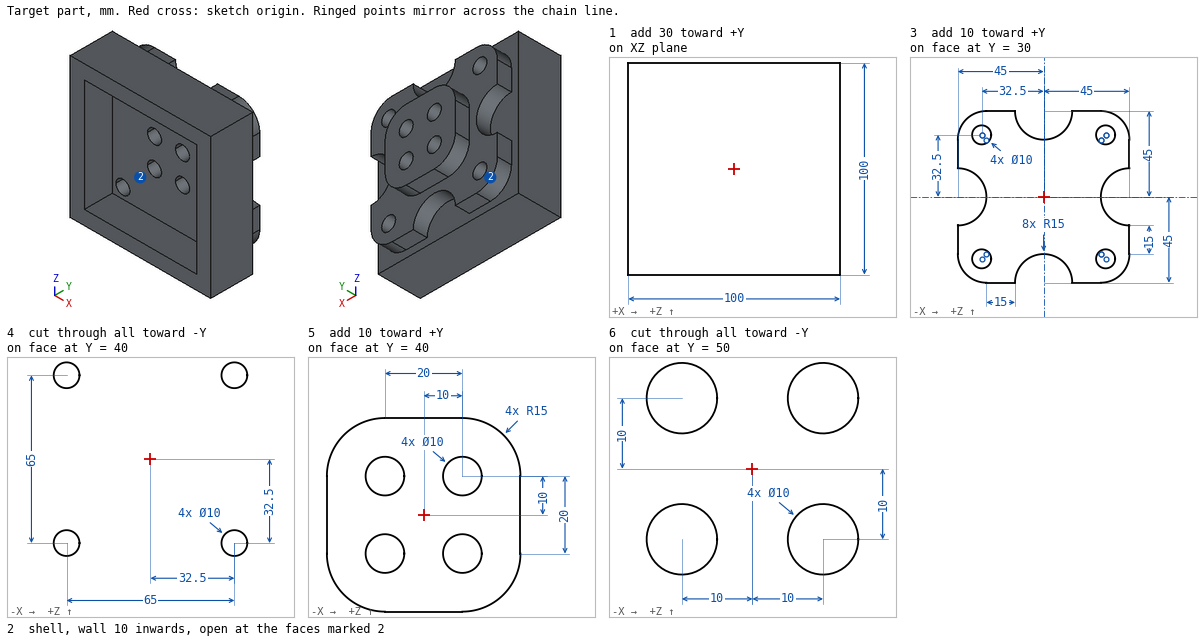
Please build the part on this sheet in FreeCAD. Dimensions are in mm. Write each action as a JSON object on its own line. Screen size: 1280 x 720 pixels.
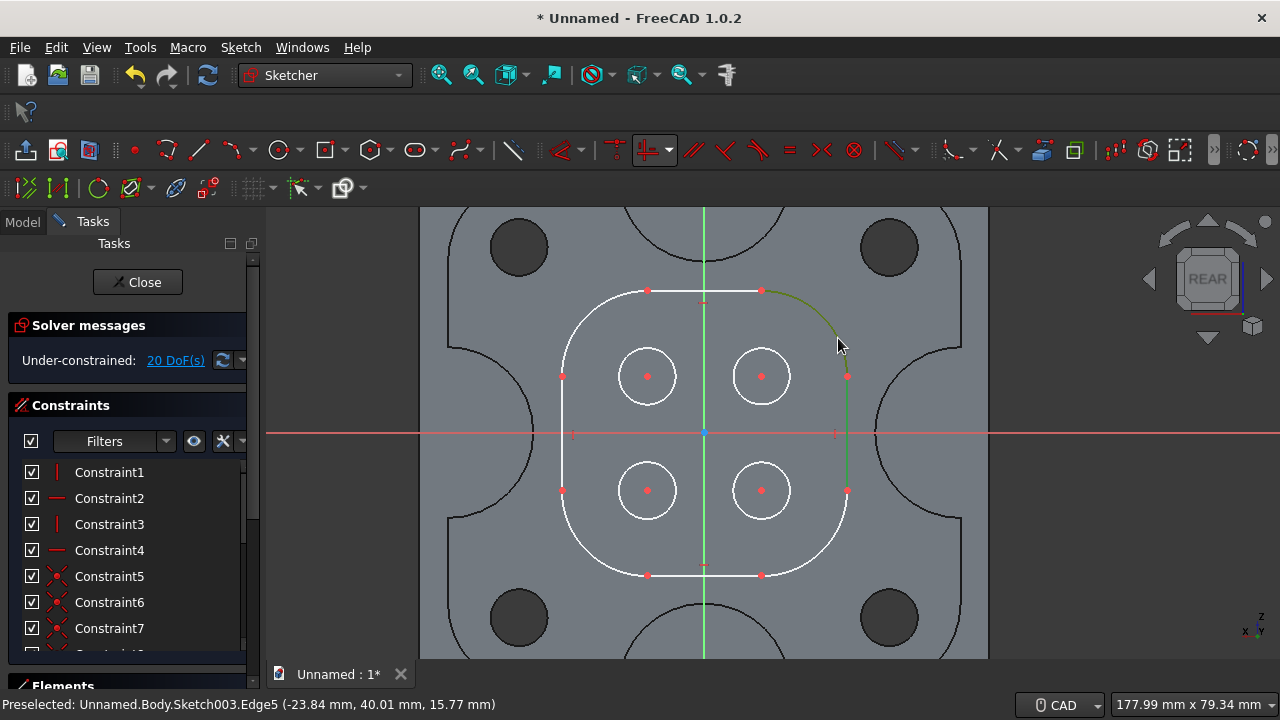
{"action": "left_click", "coordinate": [758, 150]}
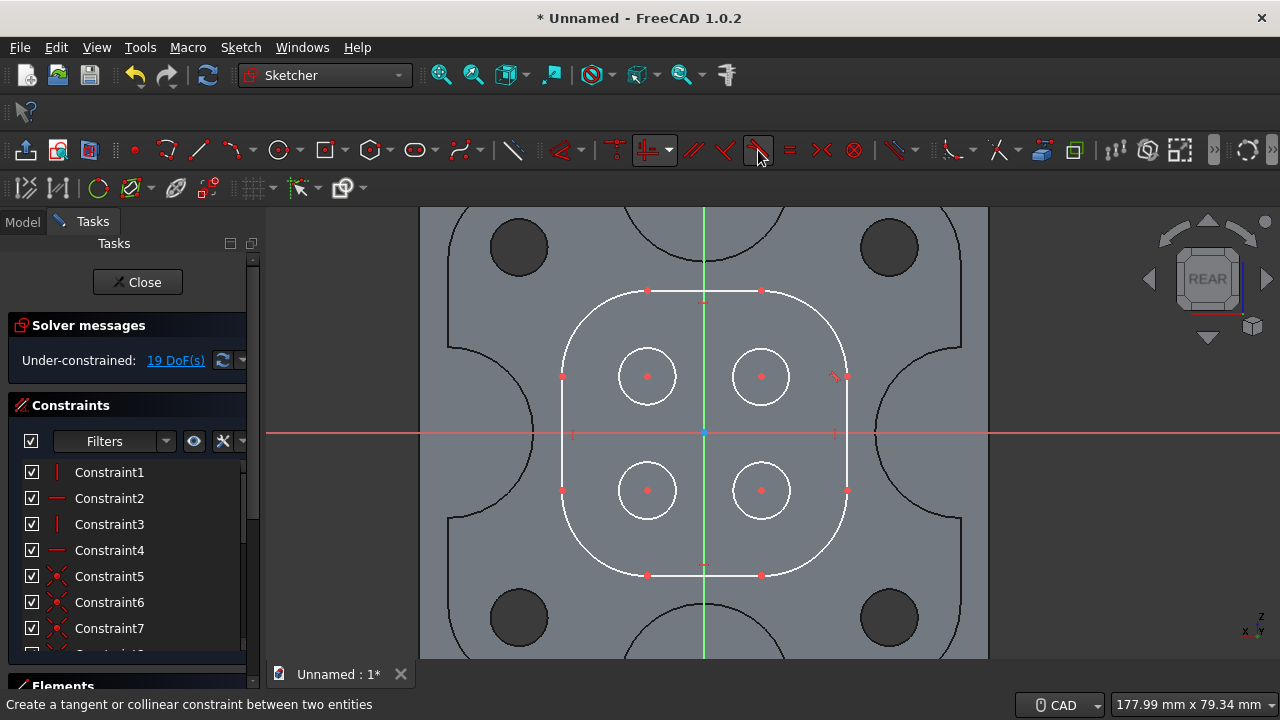
{"action": "left_click", "coordinate": [847, 457]}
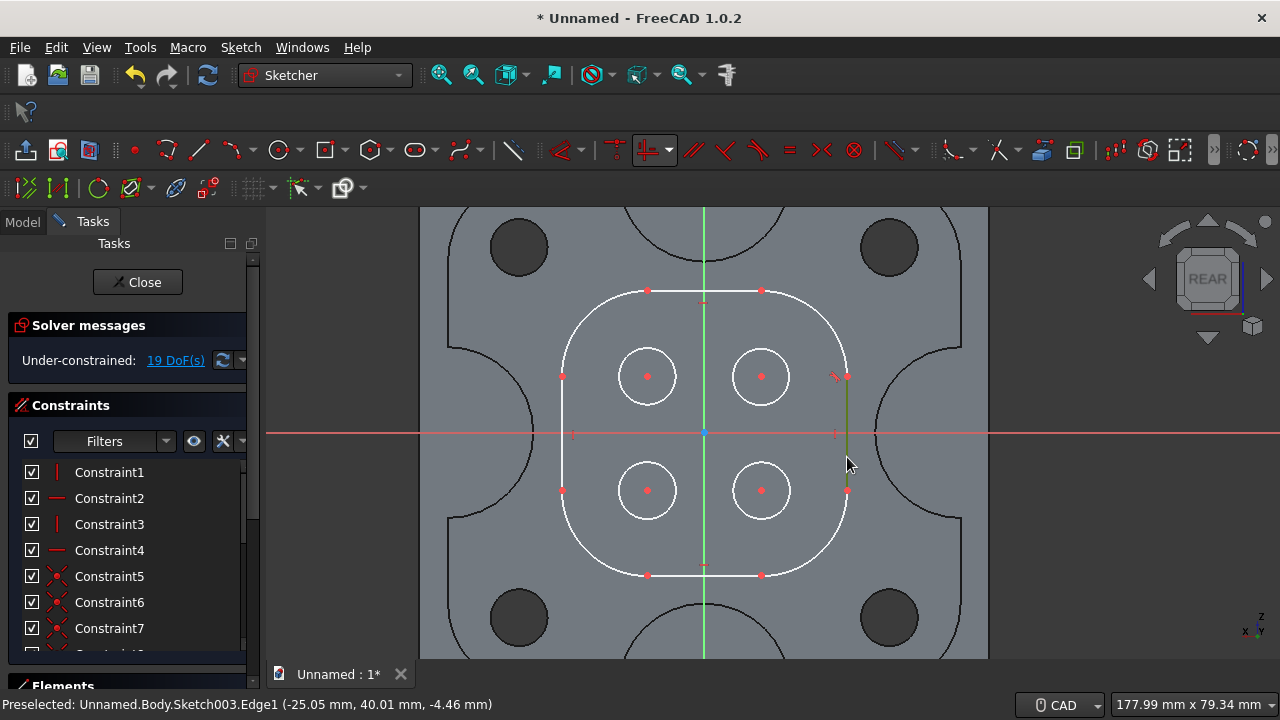
{"action": "left_click", "coordinate": [800, 567]}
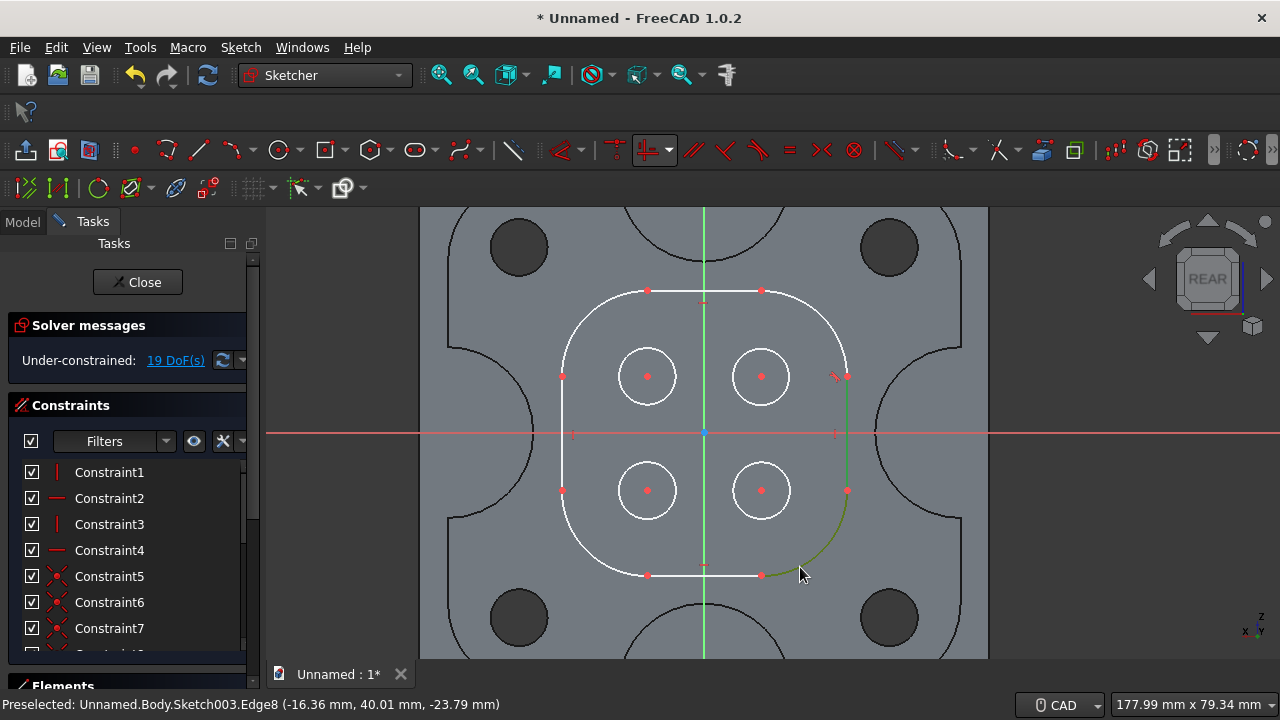
{"action": "left_click", "coordinate": [758, 150]}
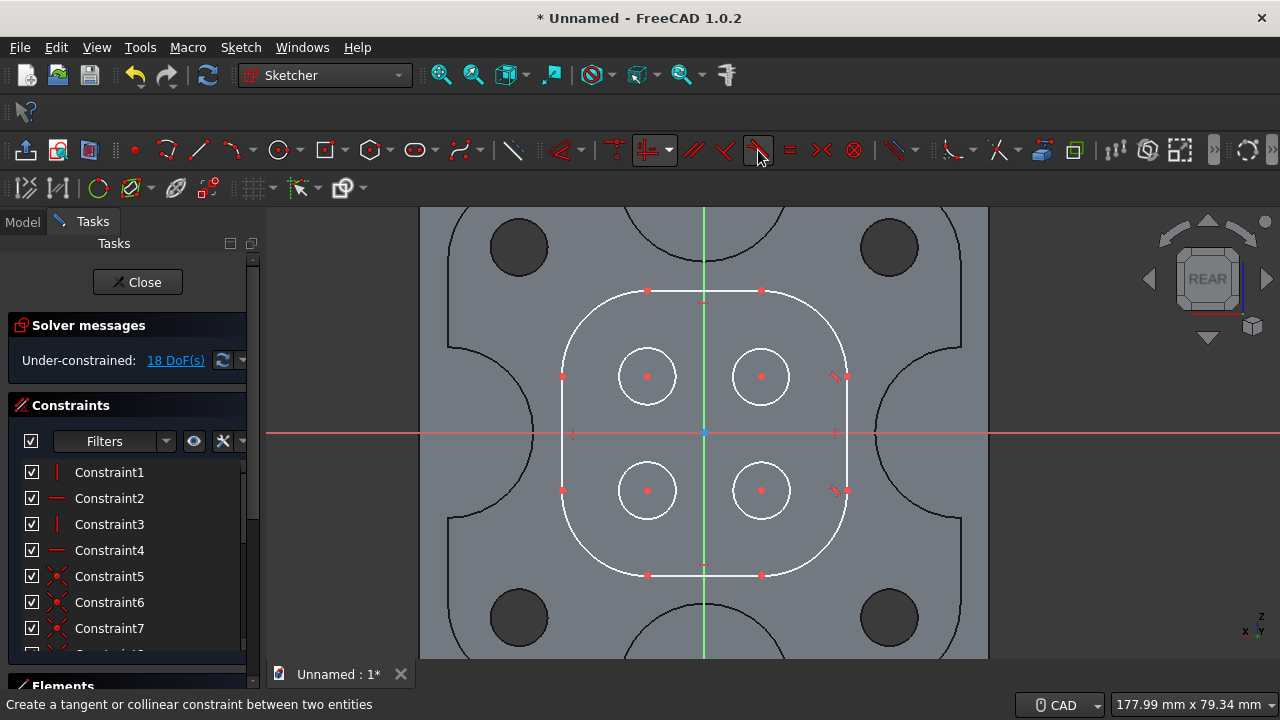
{"action": "left_click", "coordinate": [727, 291]}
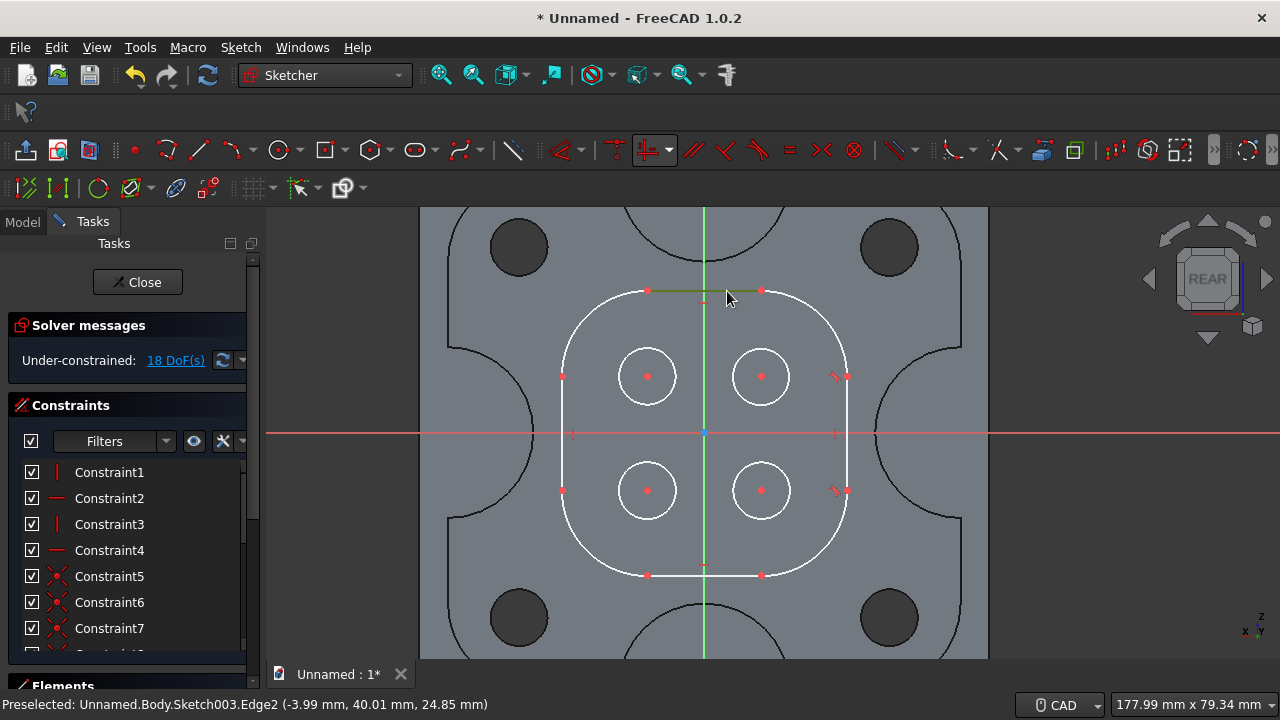
{"action": "left_click", "coordinate": [838, 338]}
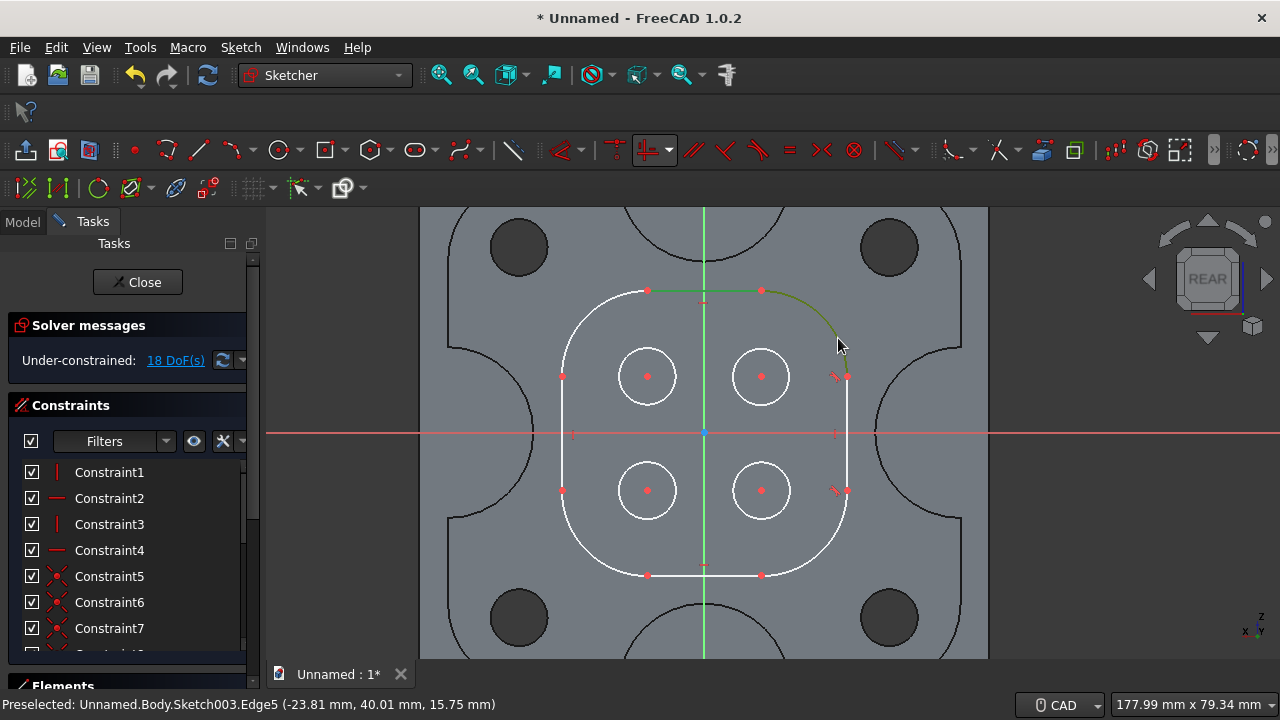
{"action": "left_click", "coordinate": [758, 150]}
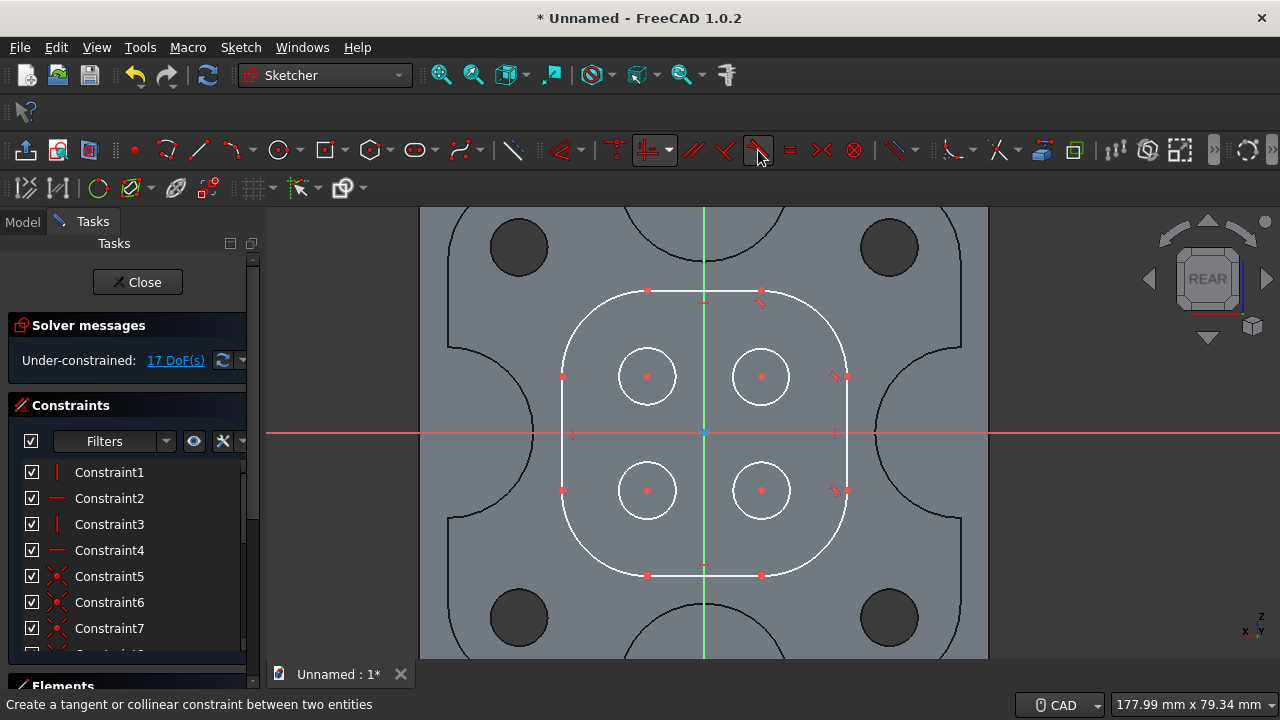
{"action": "left_click", "coordinate": [727, 291]}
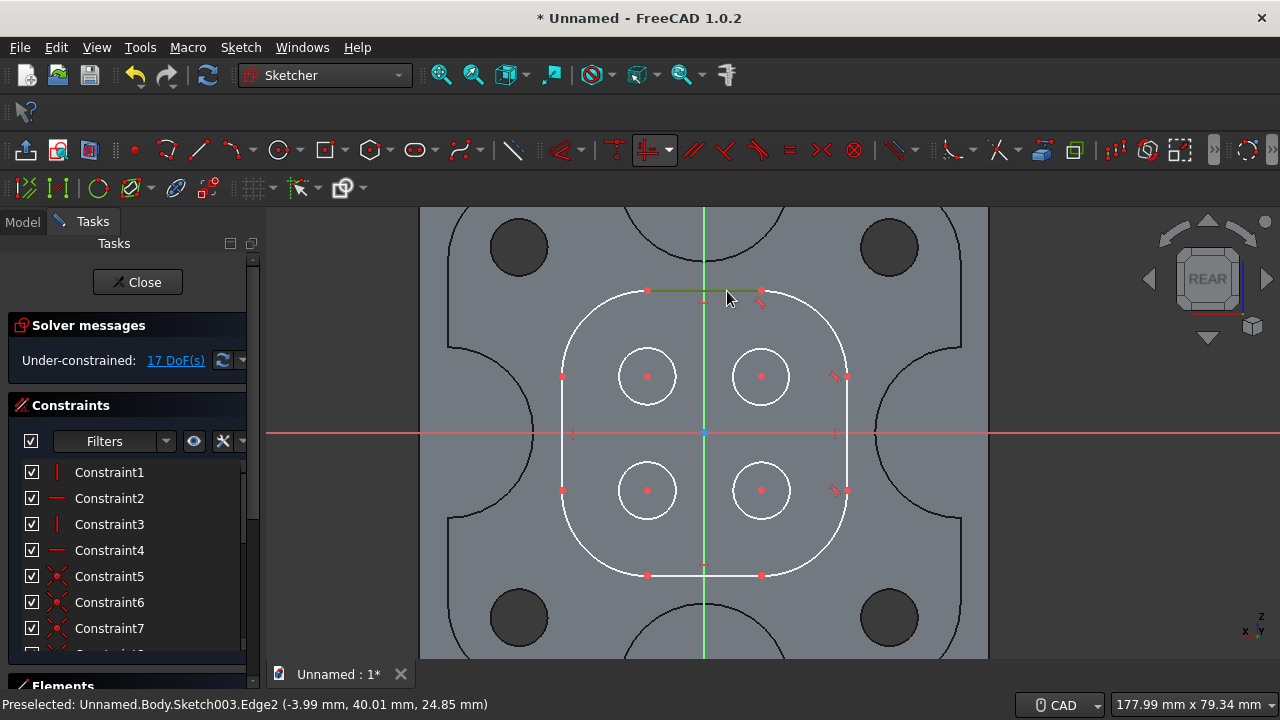
{"action": "left_click", "coordinate": [608, 301]}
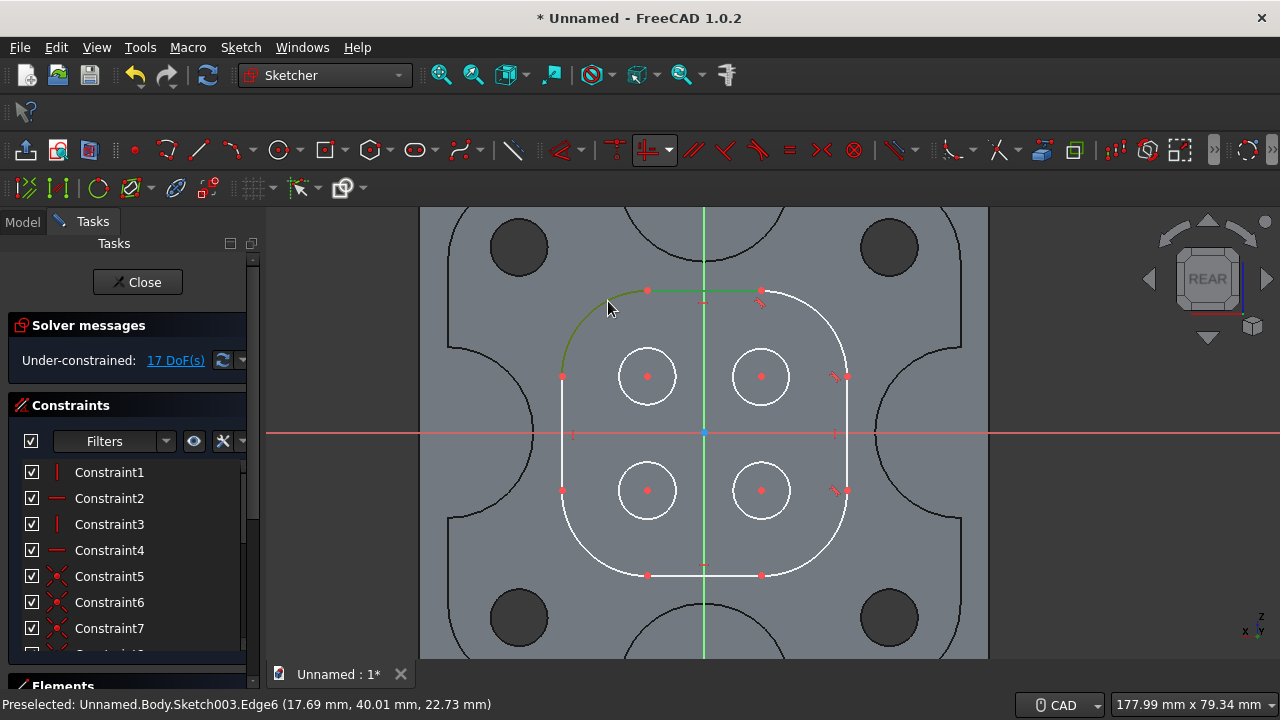
{"action": "left_click", "coordinate": [758, 150]}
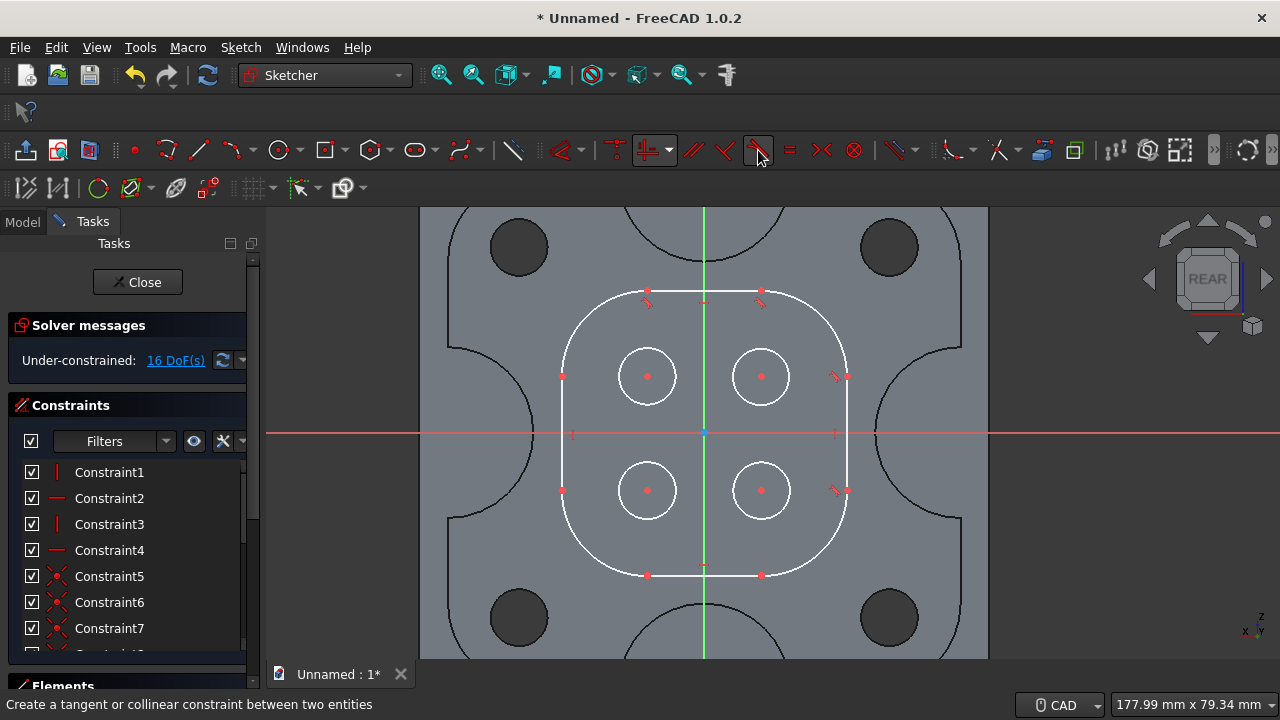
{"action": "left_click", "coordinate": [562, 411]}